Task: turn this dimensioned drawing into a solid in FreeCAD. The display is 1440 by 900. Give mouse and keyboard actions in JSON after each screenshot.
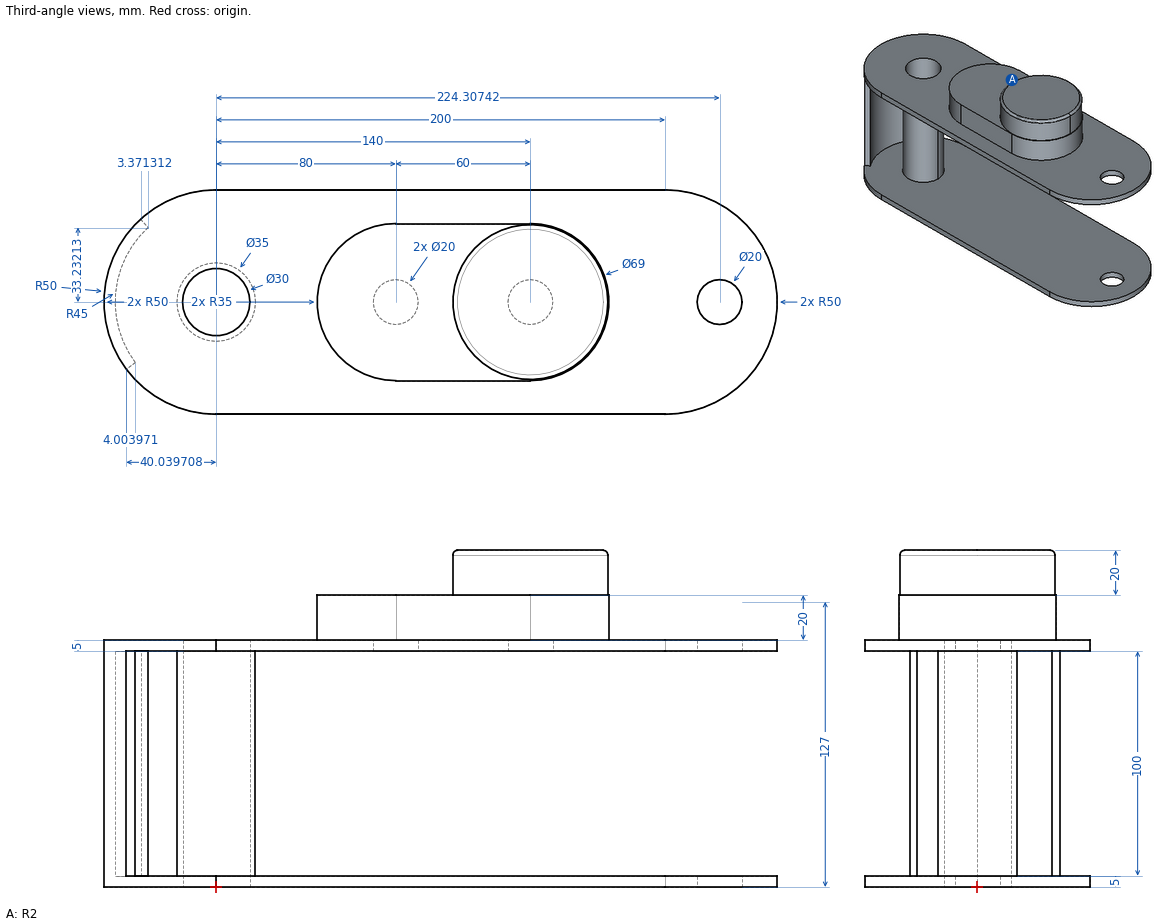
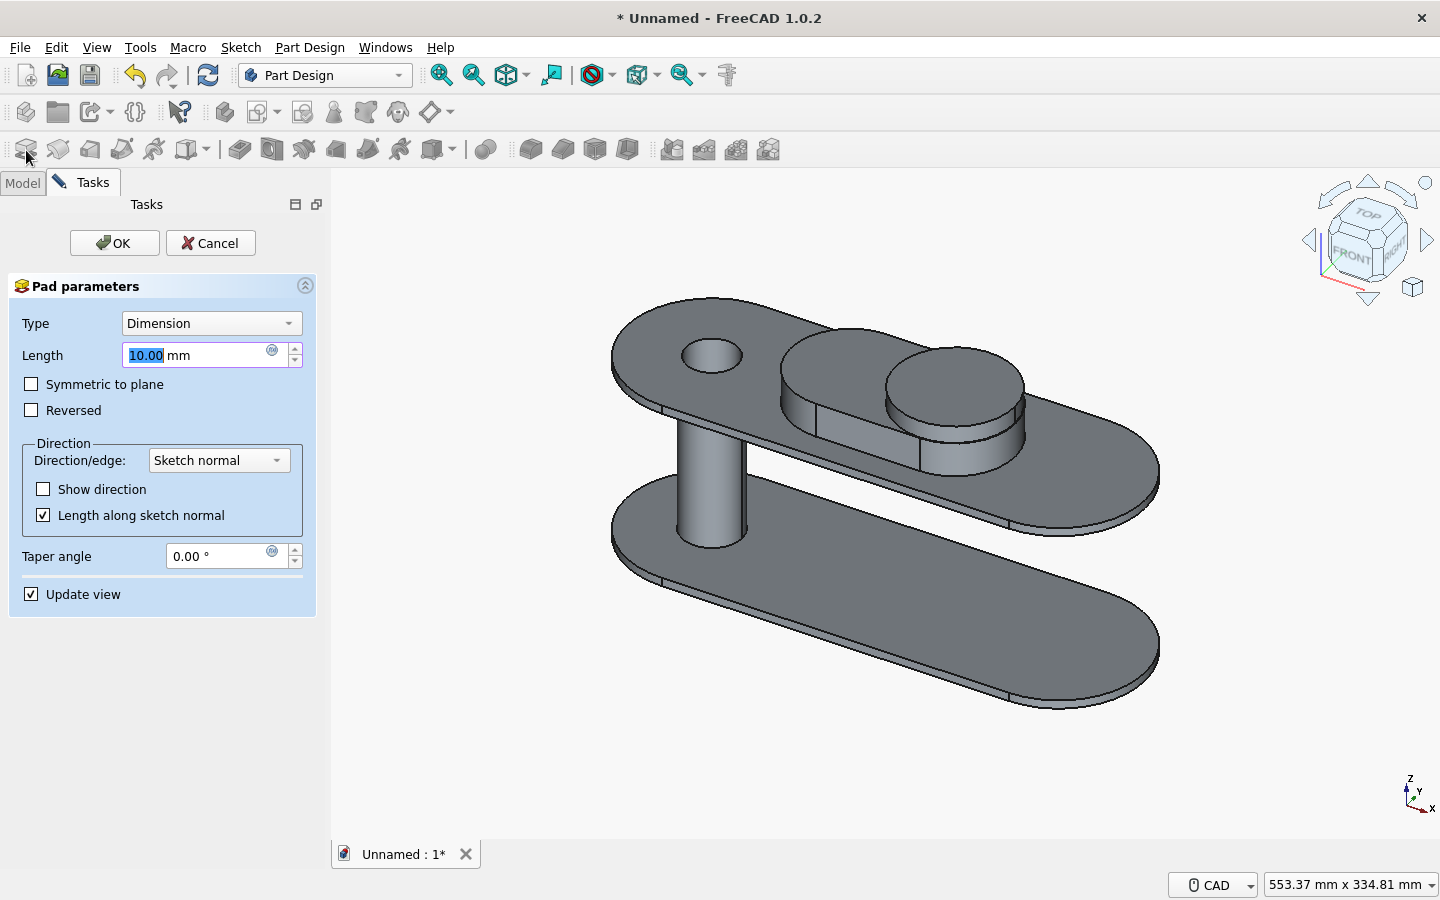
{"action": "type", "text": "20"}
{"action": "key", "text": "Tab"}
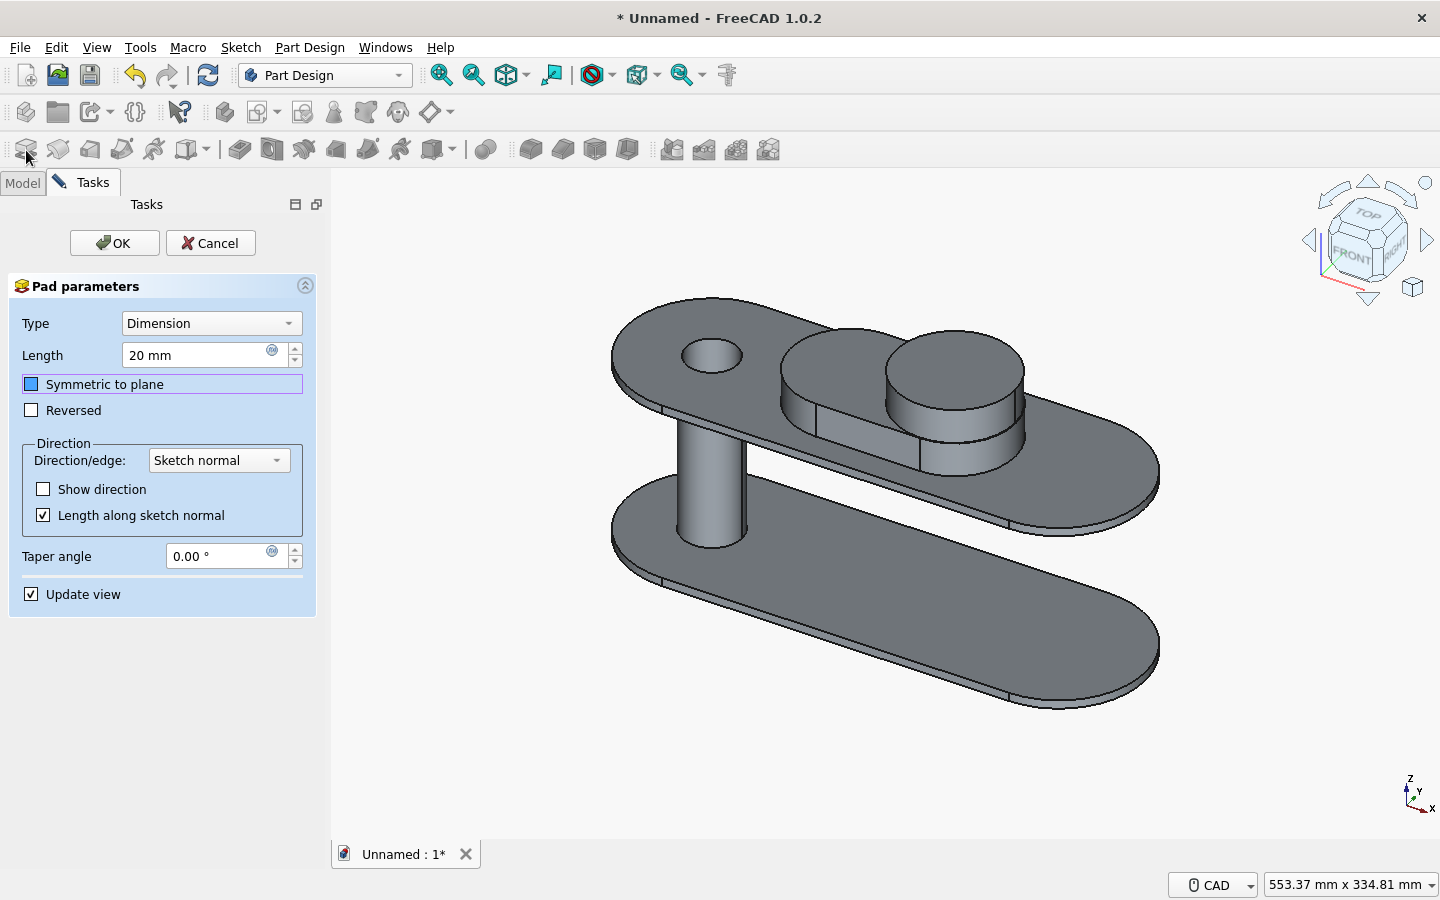
{"action": "left_click", "coordinate": [115, 243]}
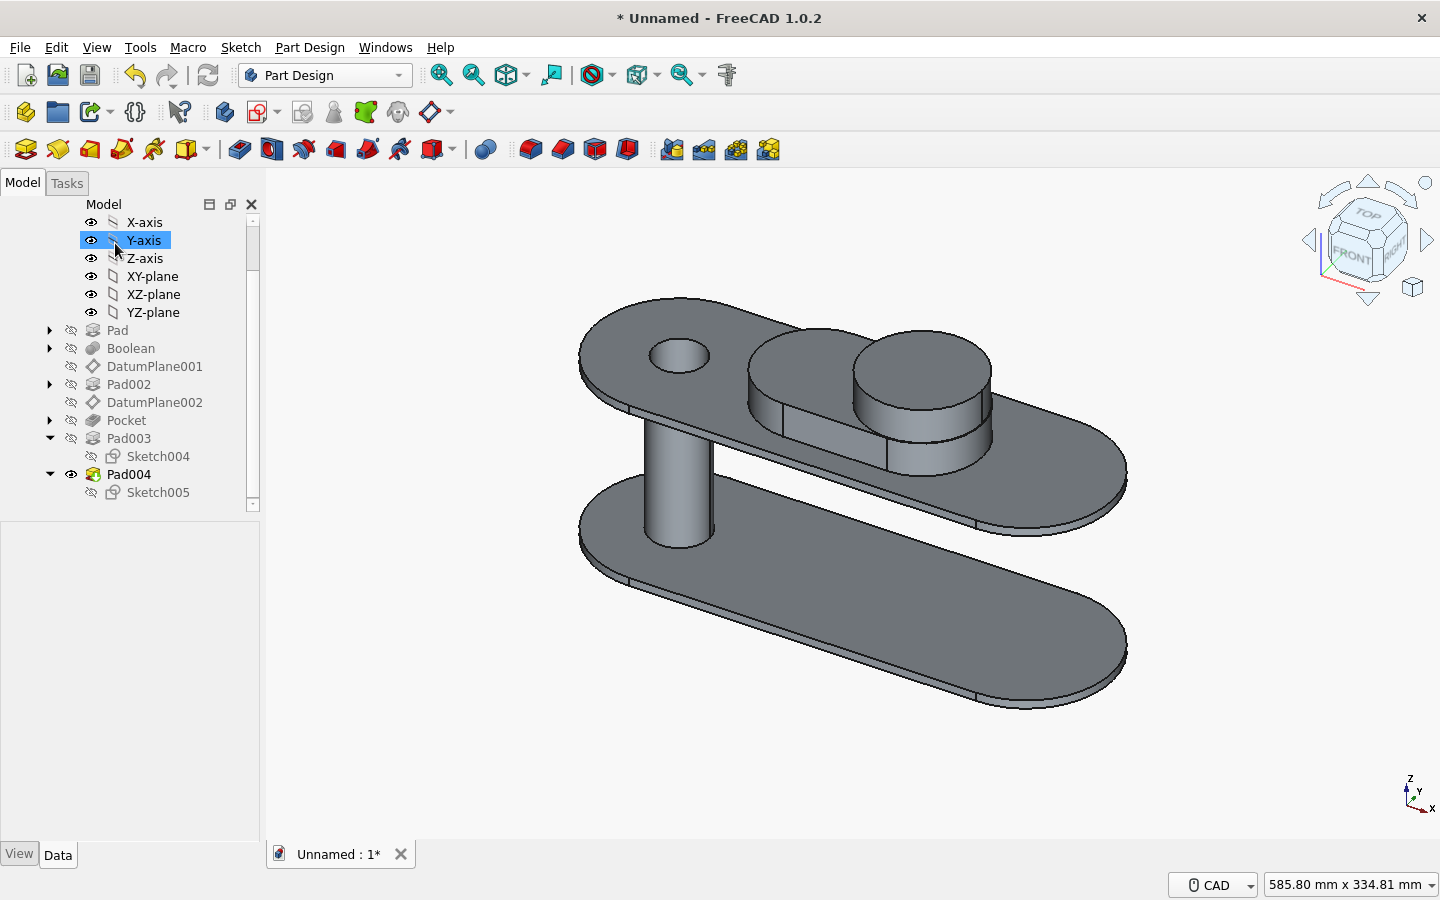
{"action": "key", "text": "5"}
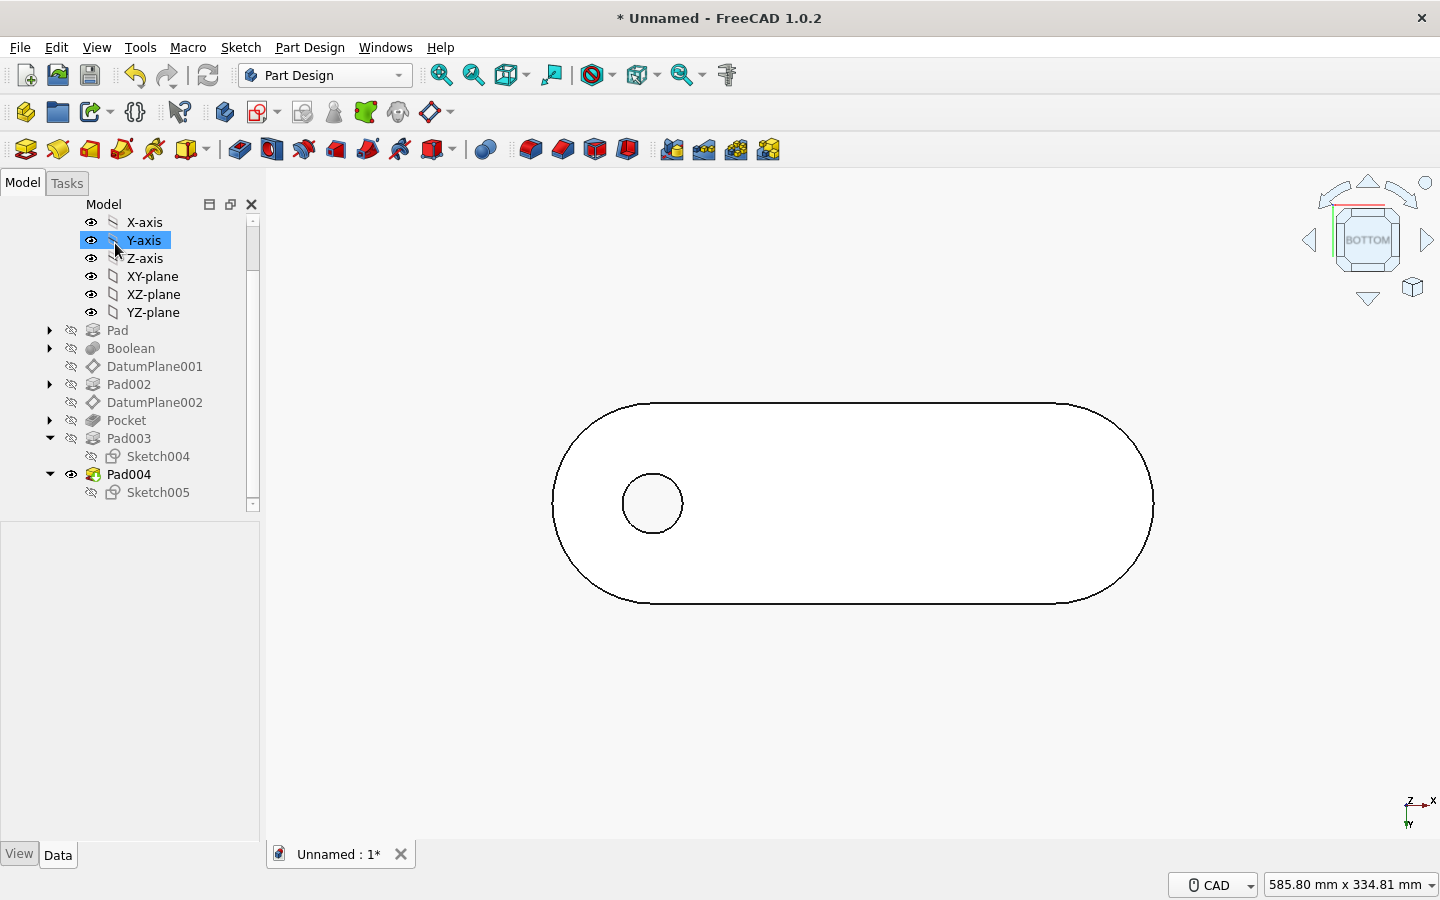
{"action": "left_click", "coordinate": [1025, 502]}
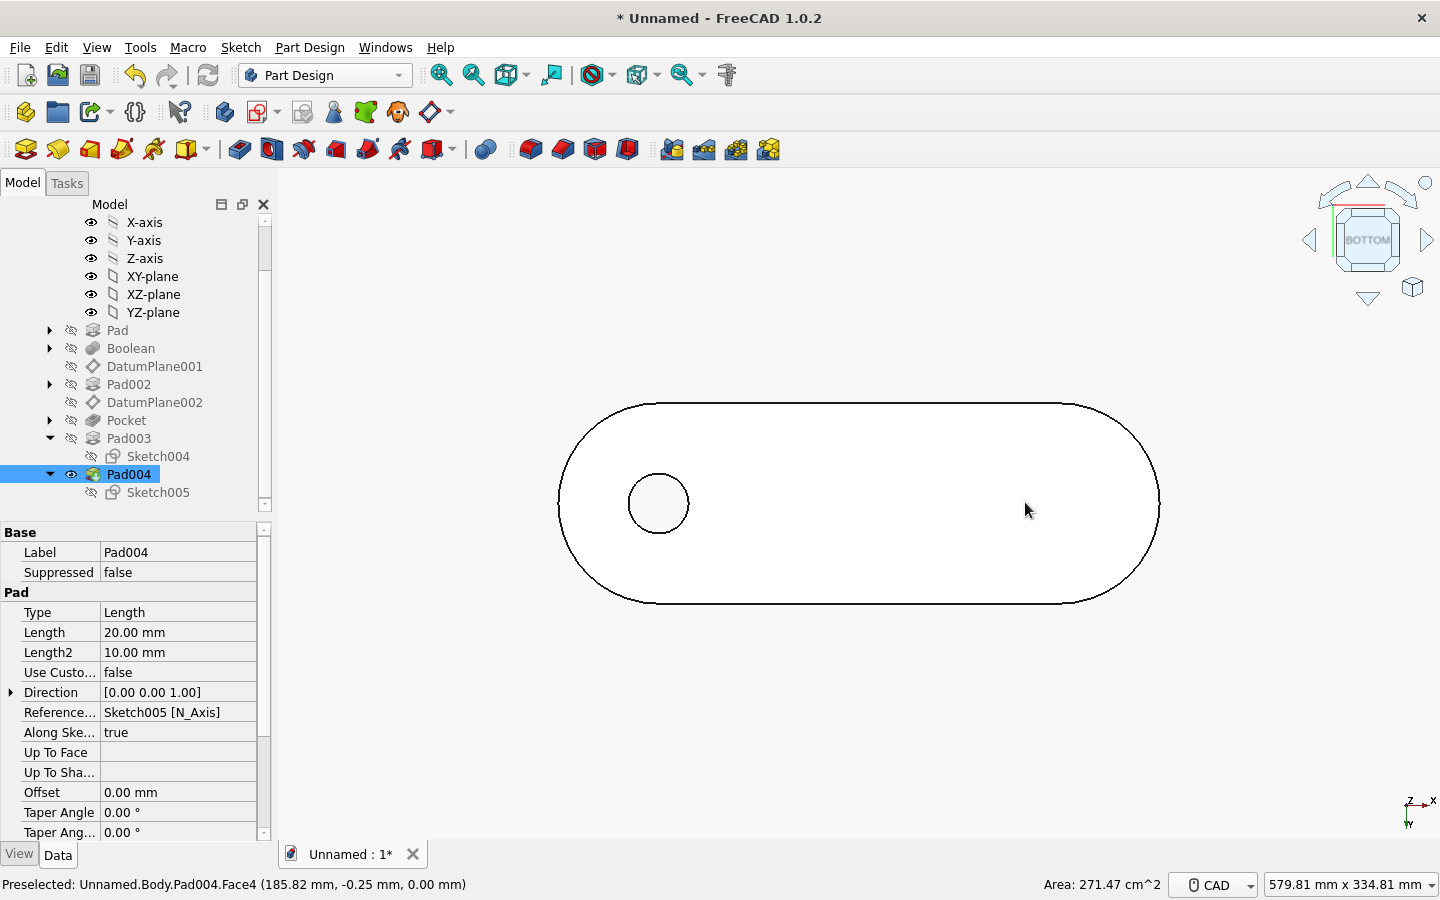
{"action": "left_click", "coordinate": [258, 112]}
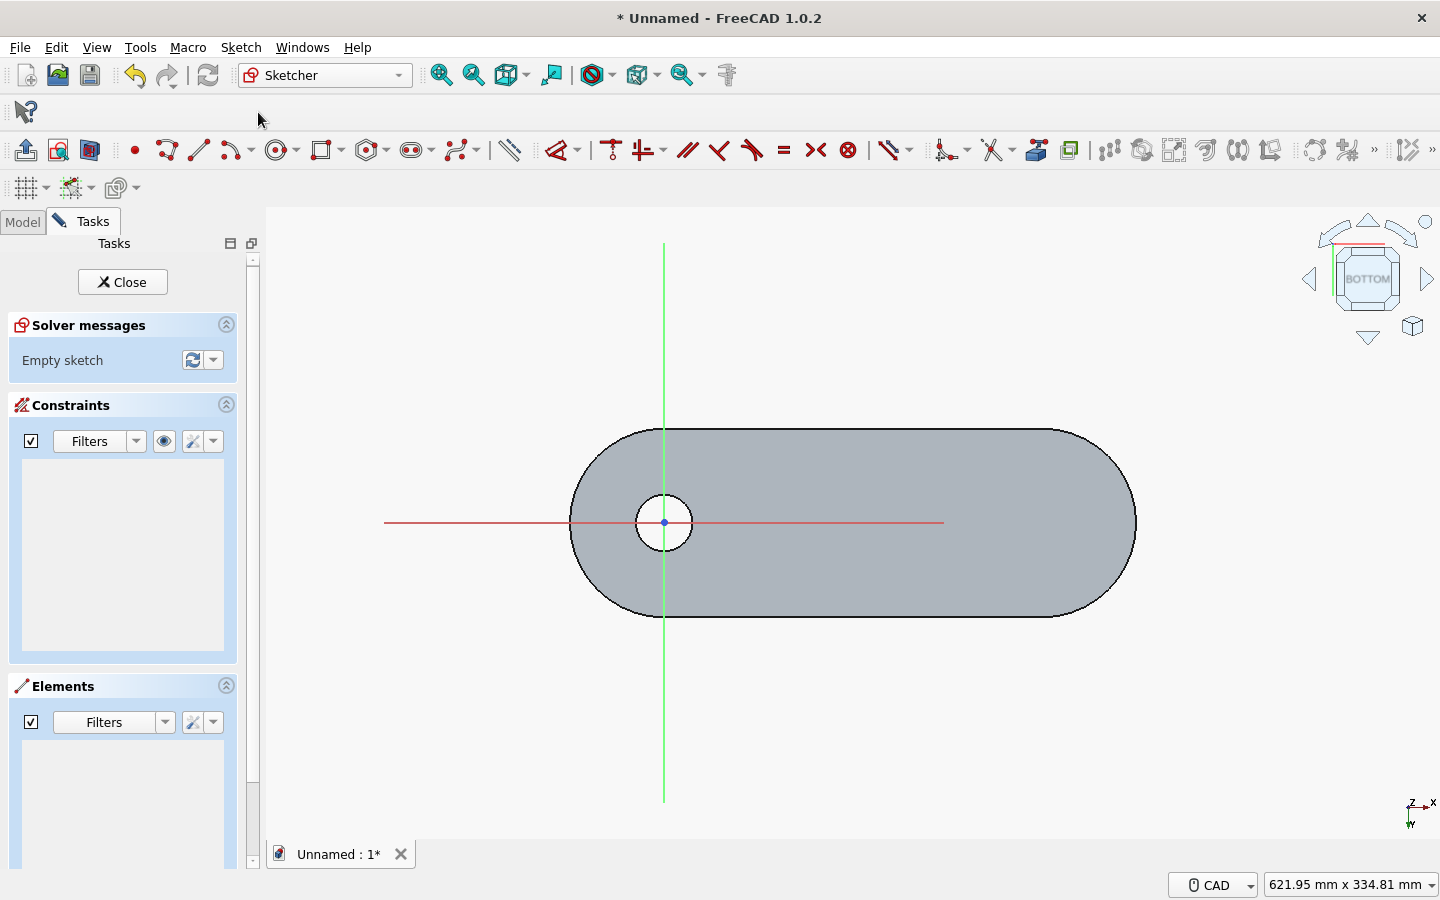
{"action": "scroll", "coordinate": [1118, 523], "scroll_direction": "up", "scroll_amount": 12}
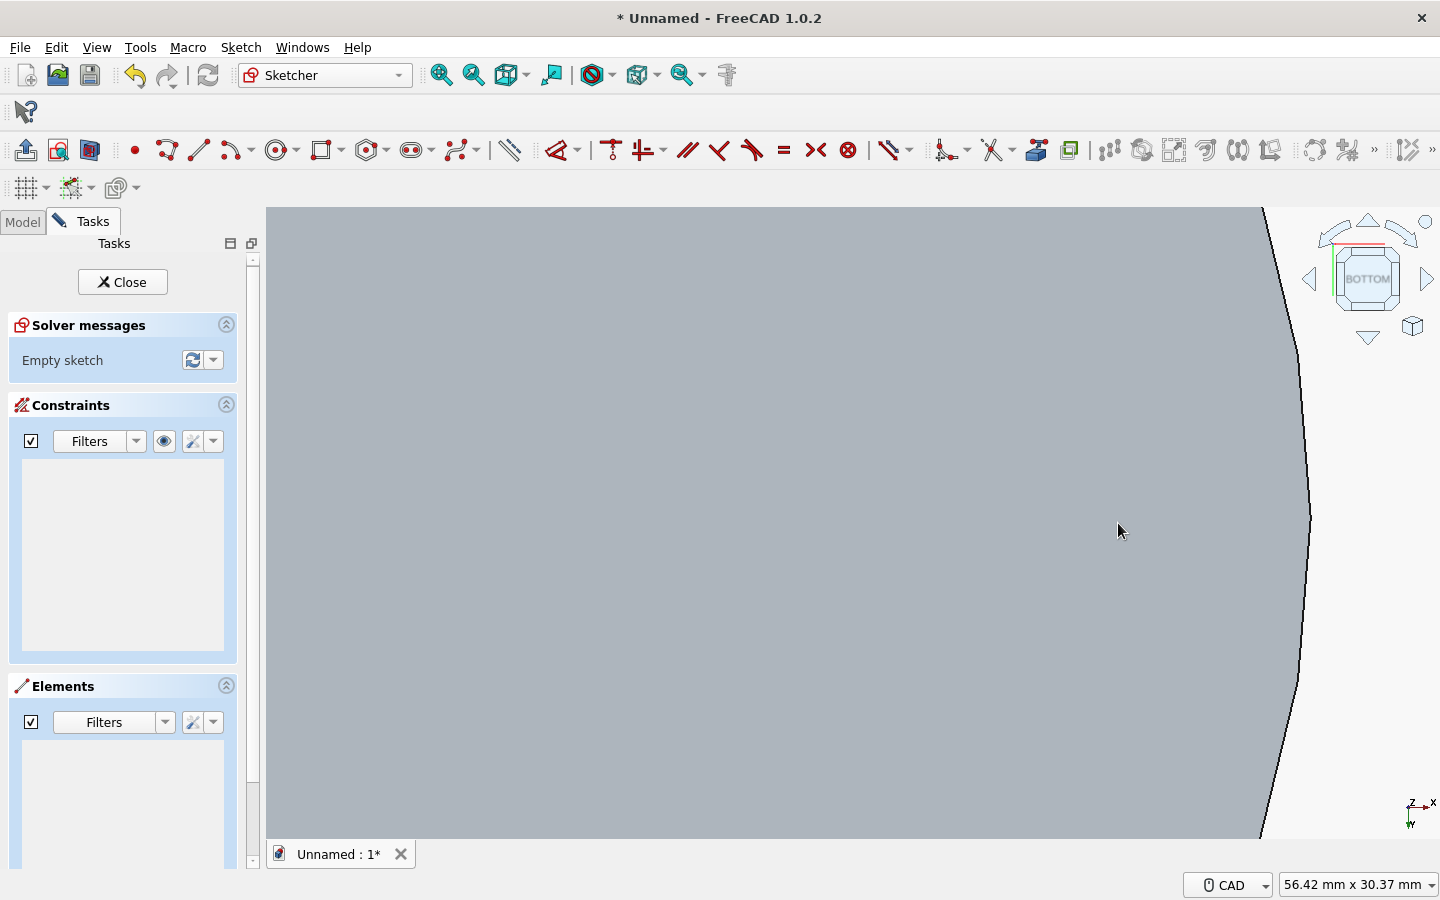
{"action": "left_click", "coordinate": [276, 150]}